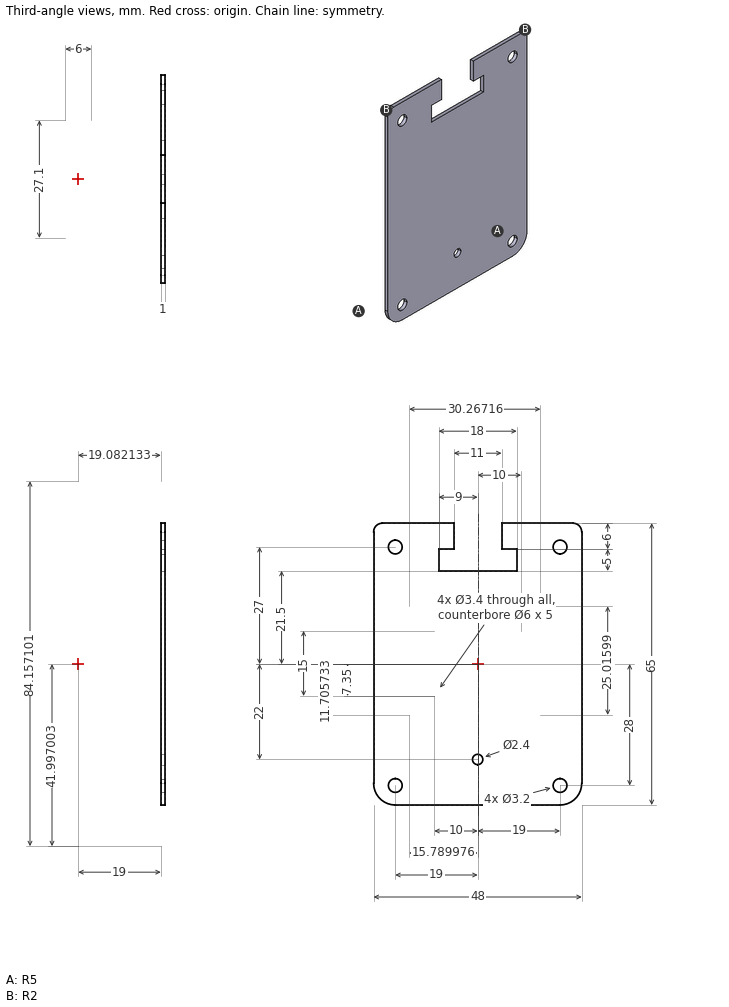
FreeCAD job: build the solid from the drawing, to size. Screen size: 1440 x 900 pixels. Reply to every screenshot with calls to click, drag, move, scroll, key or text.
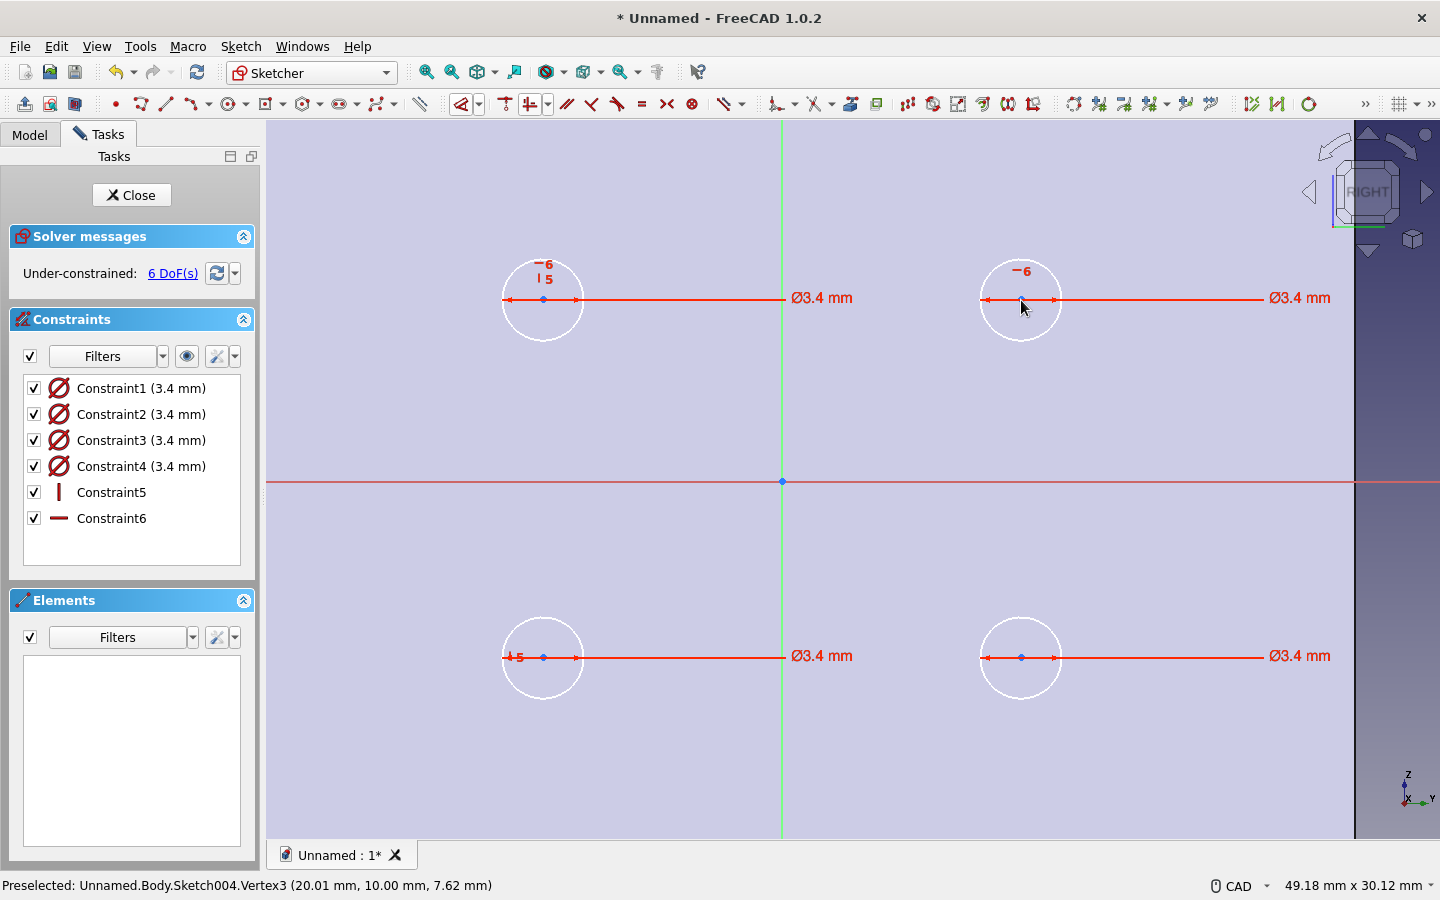
click(1021, 300)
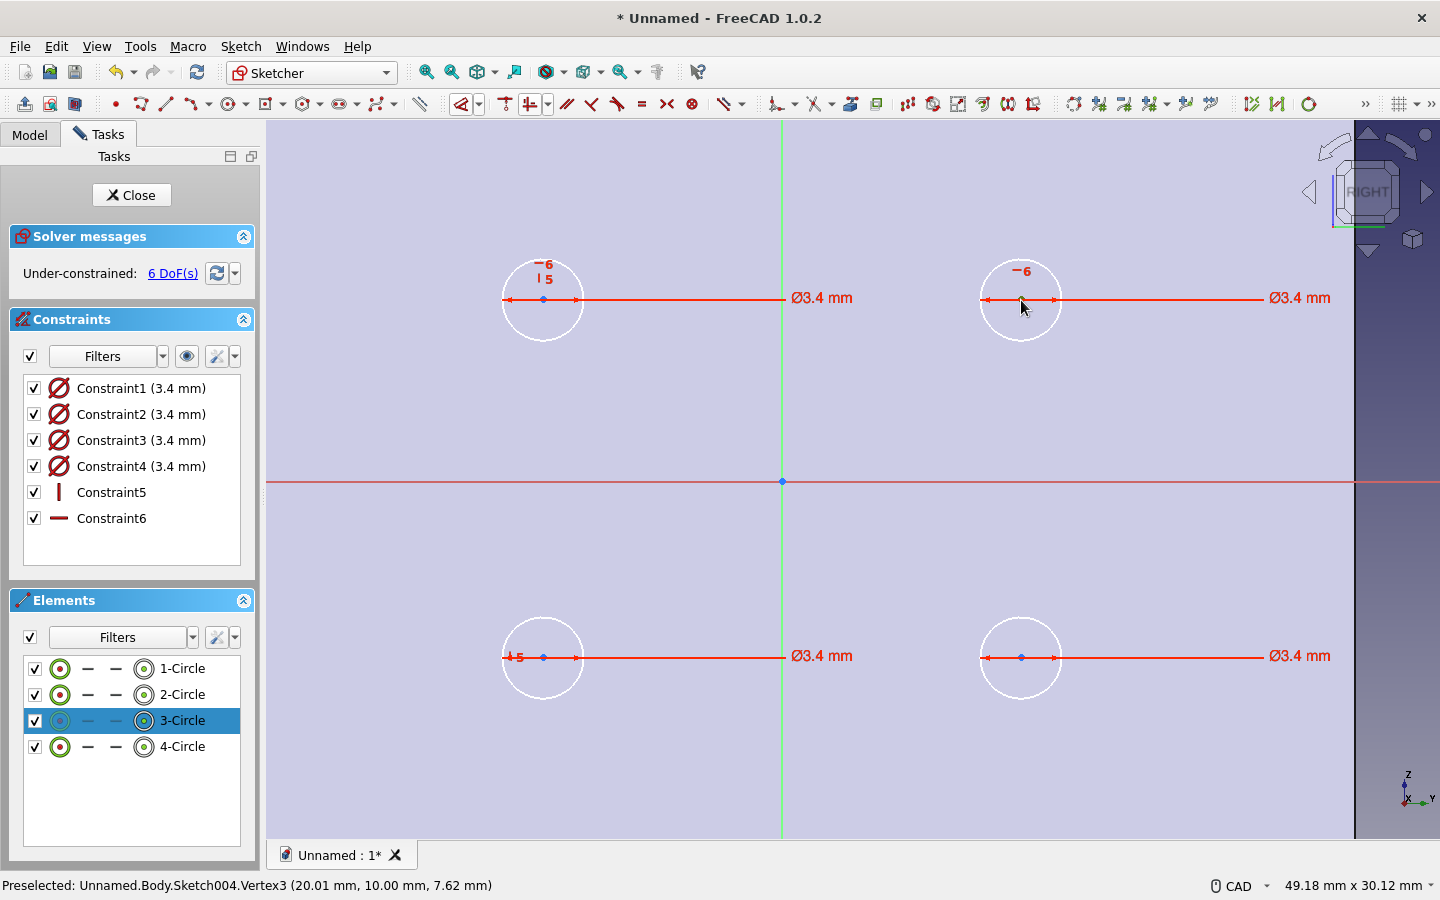
click(1021, 658)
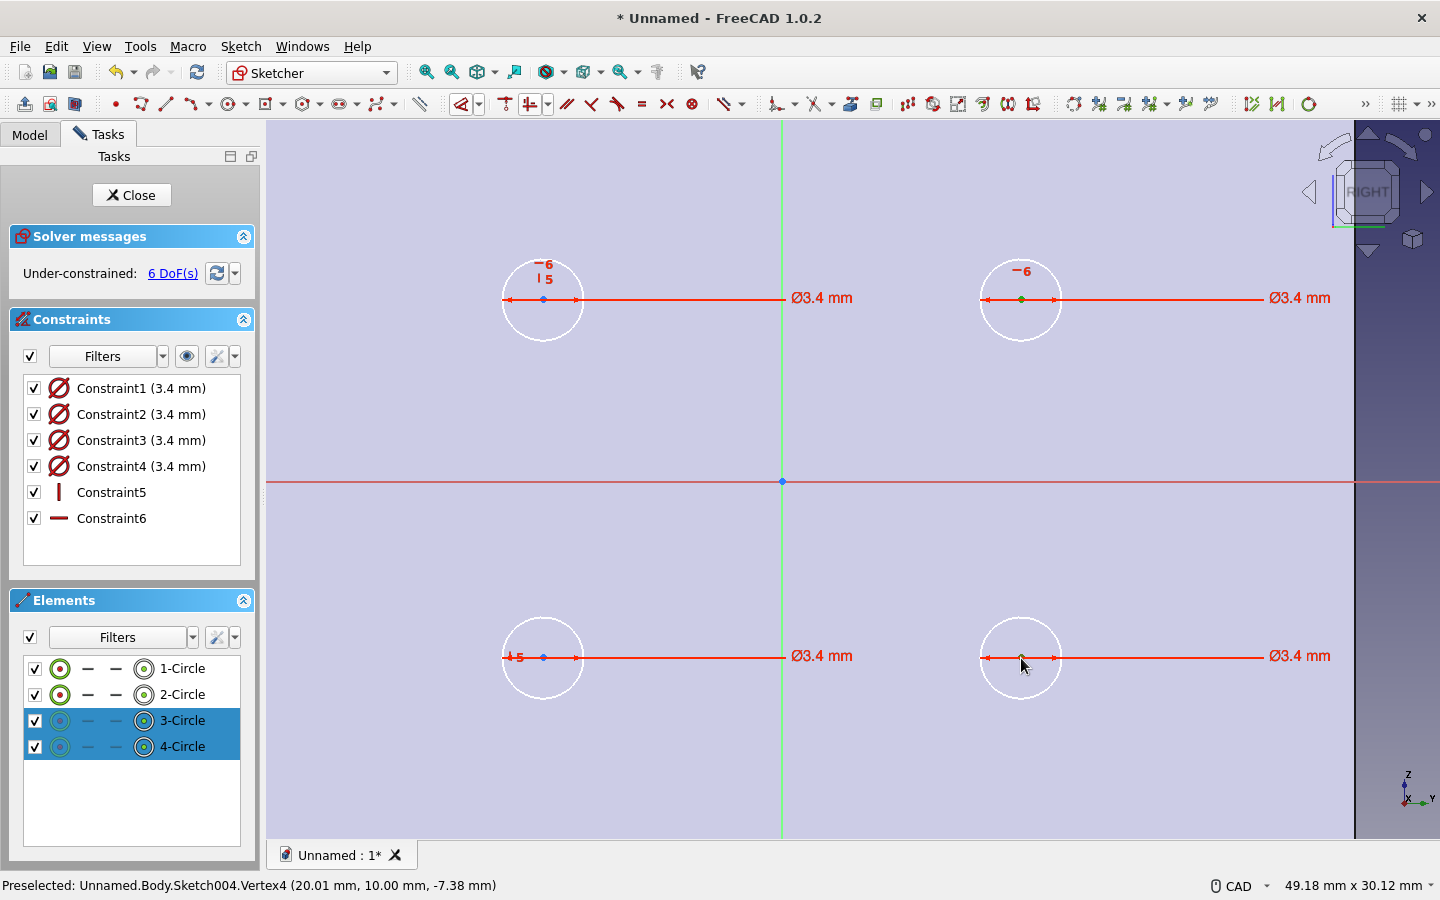
key(v)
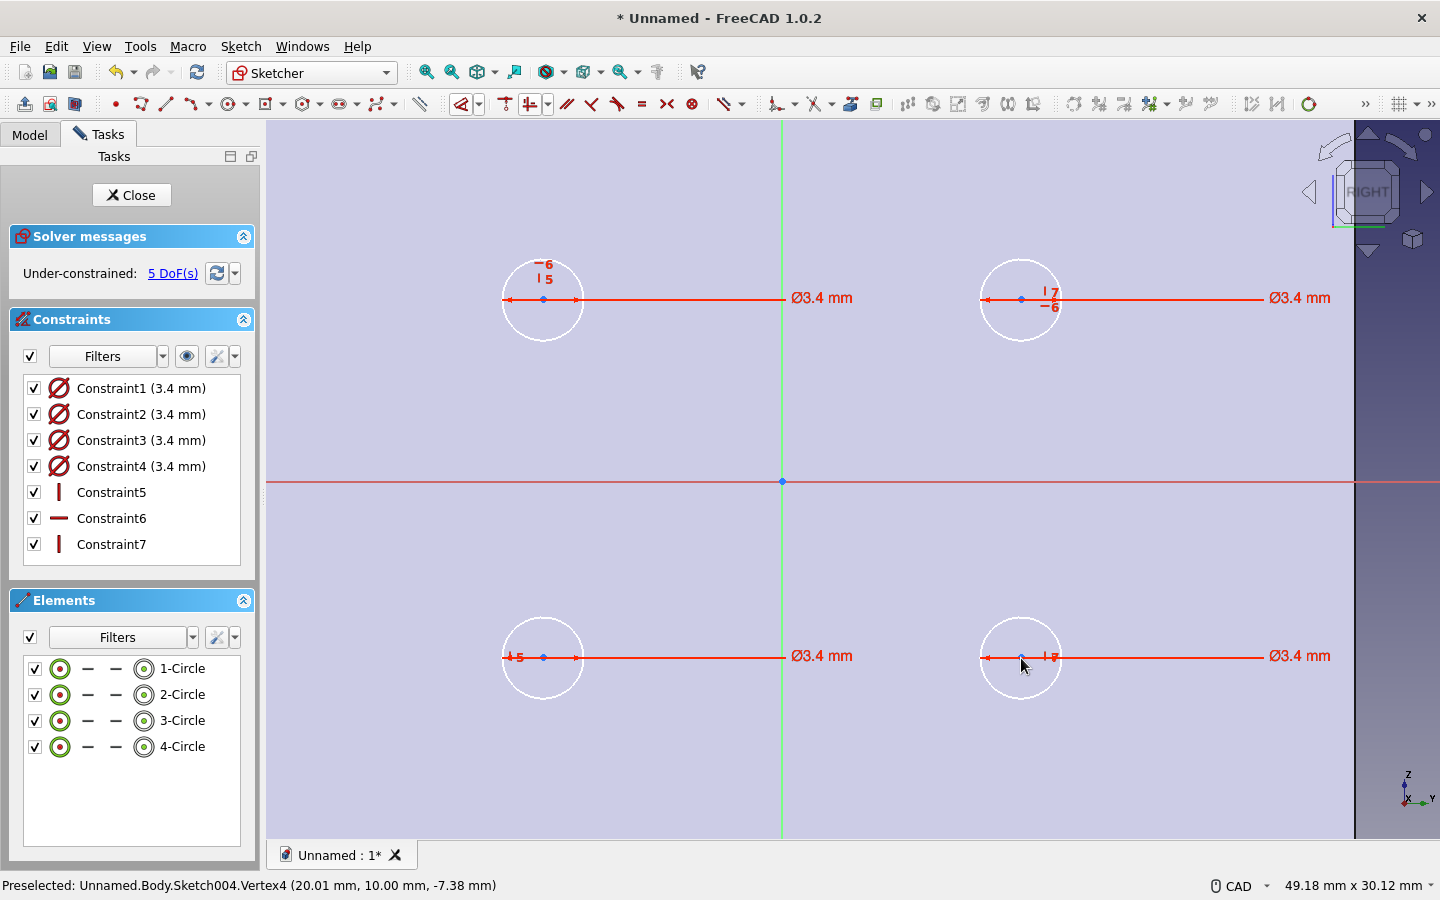
click(543, 658)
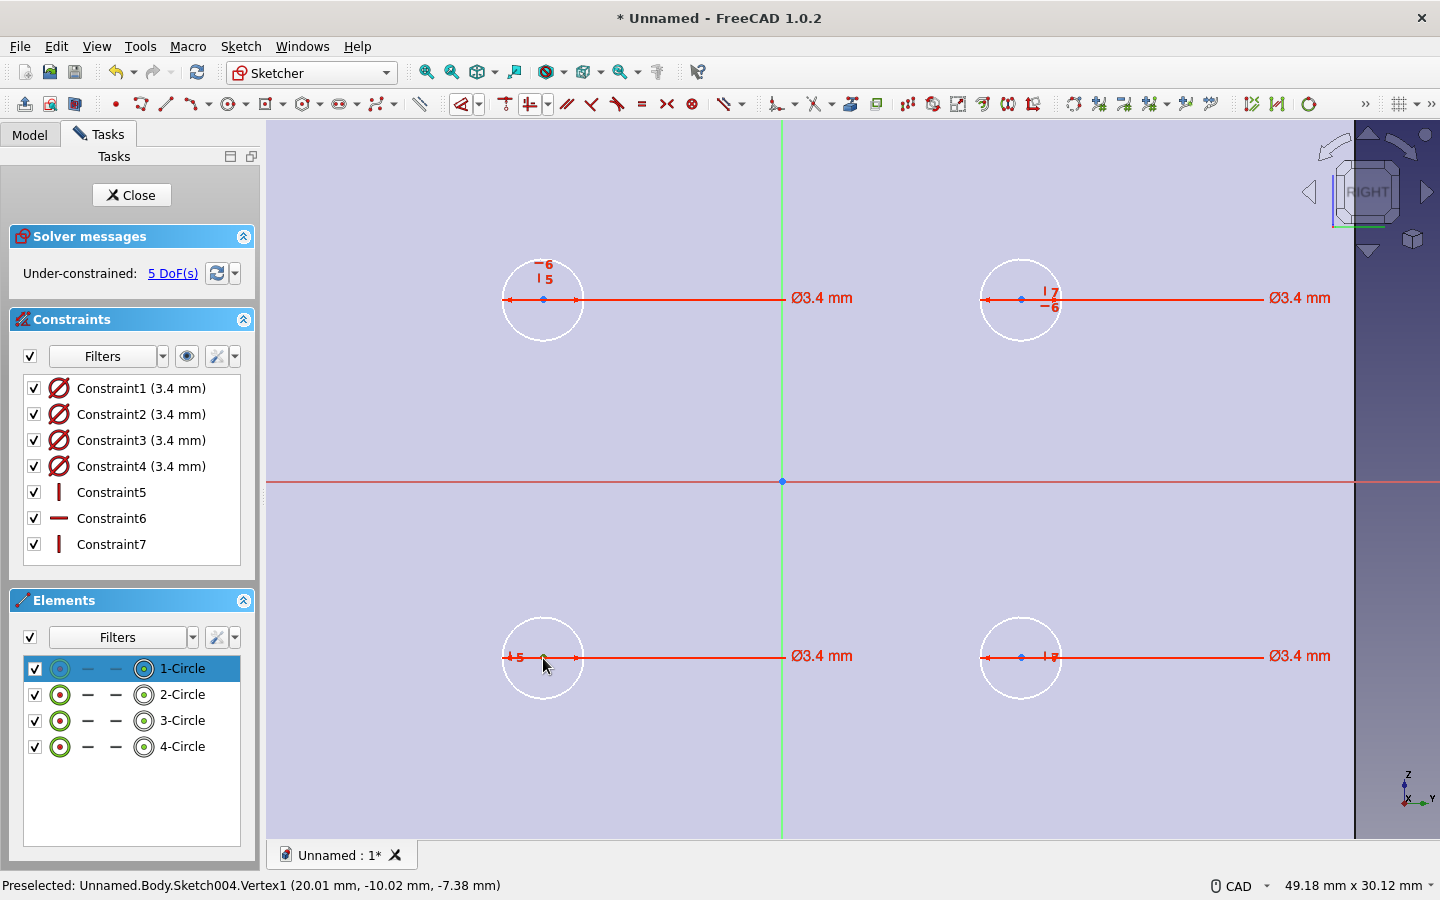
click(1021, 658)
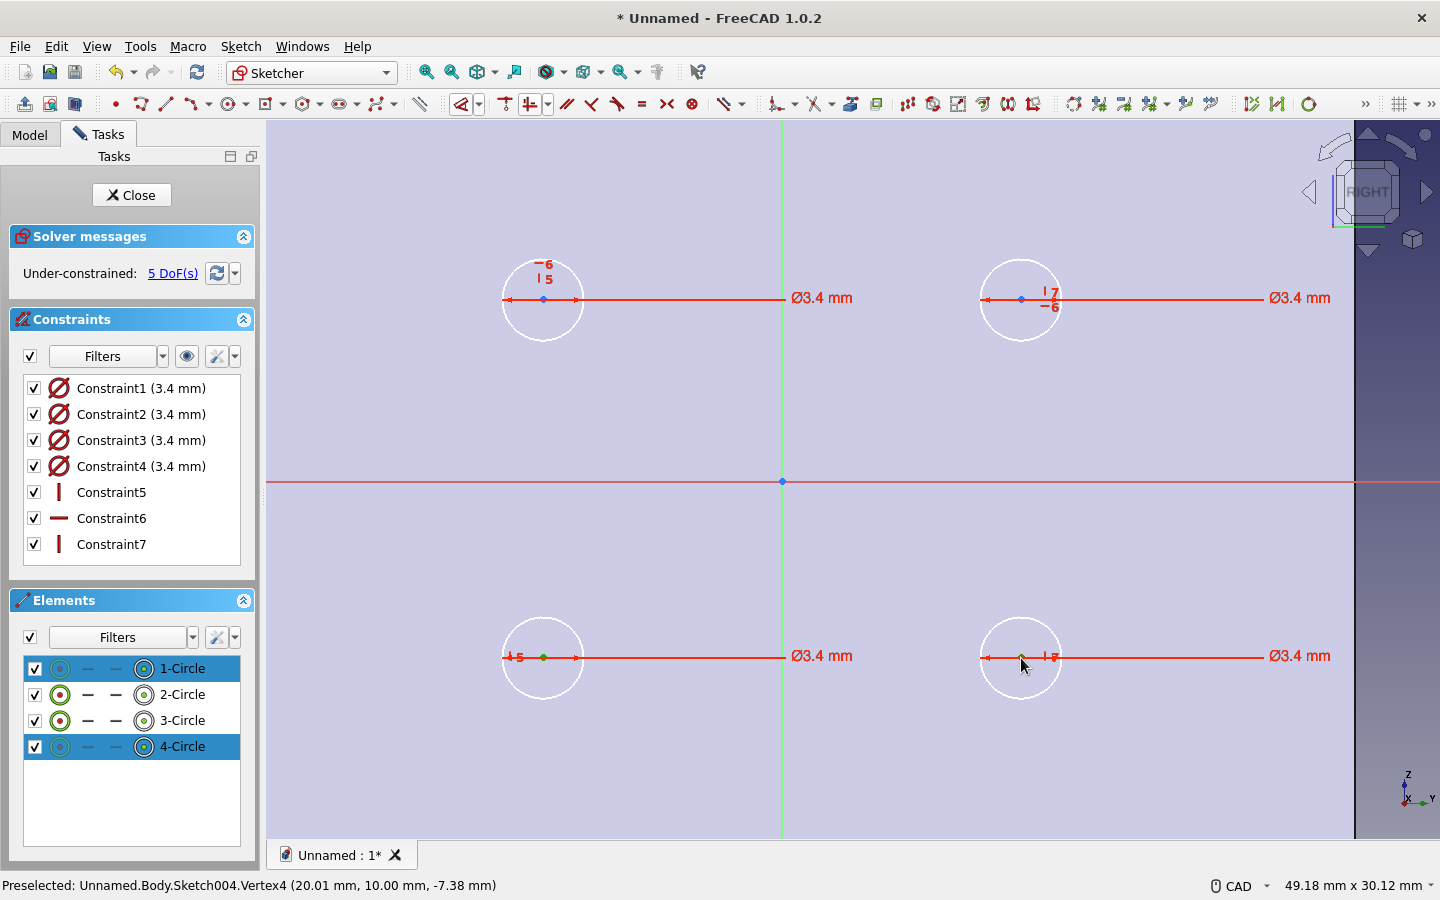
key(h)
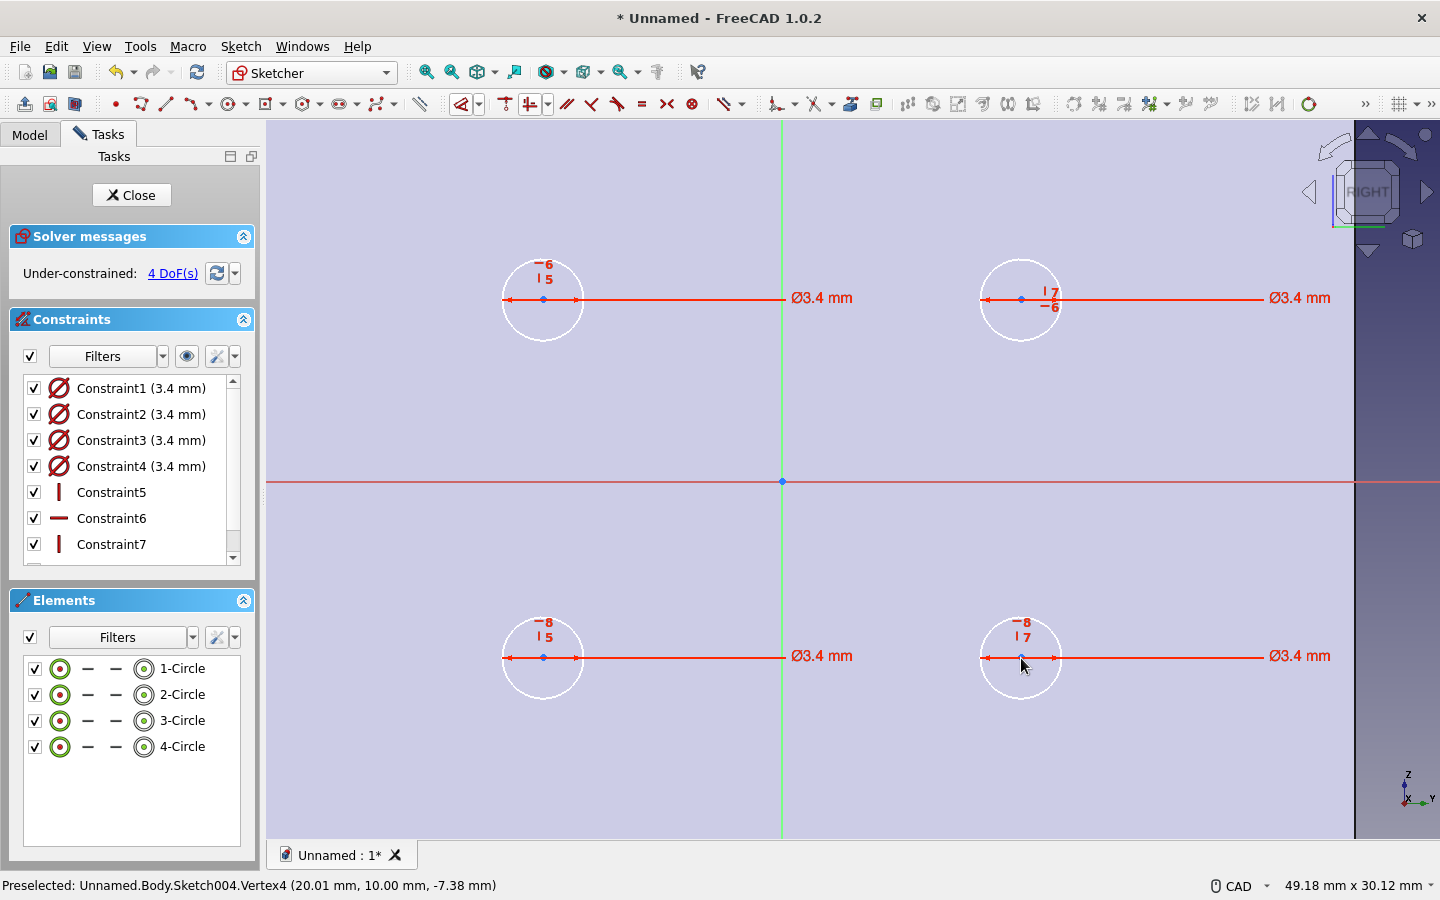
click(543, 658)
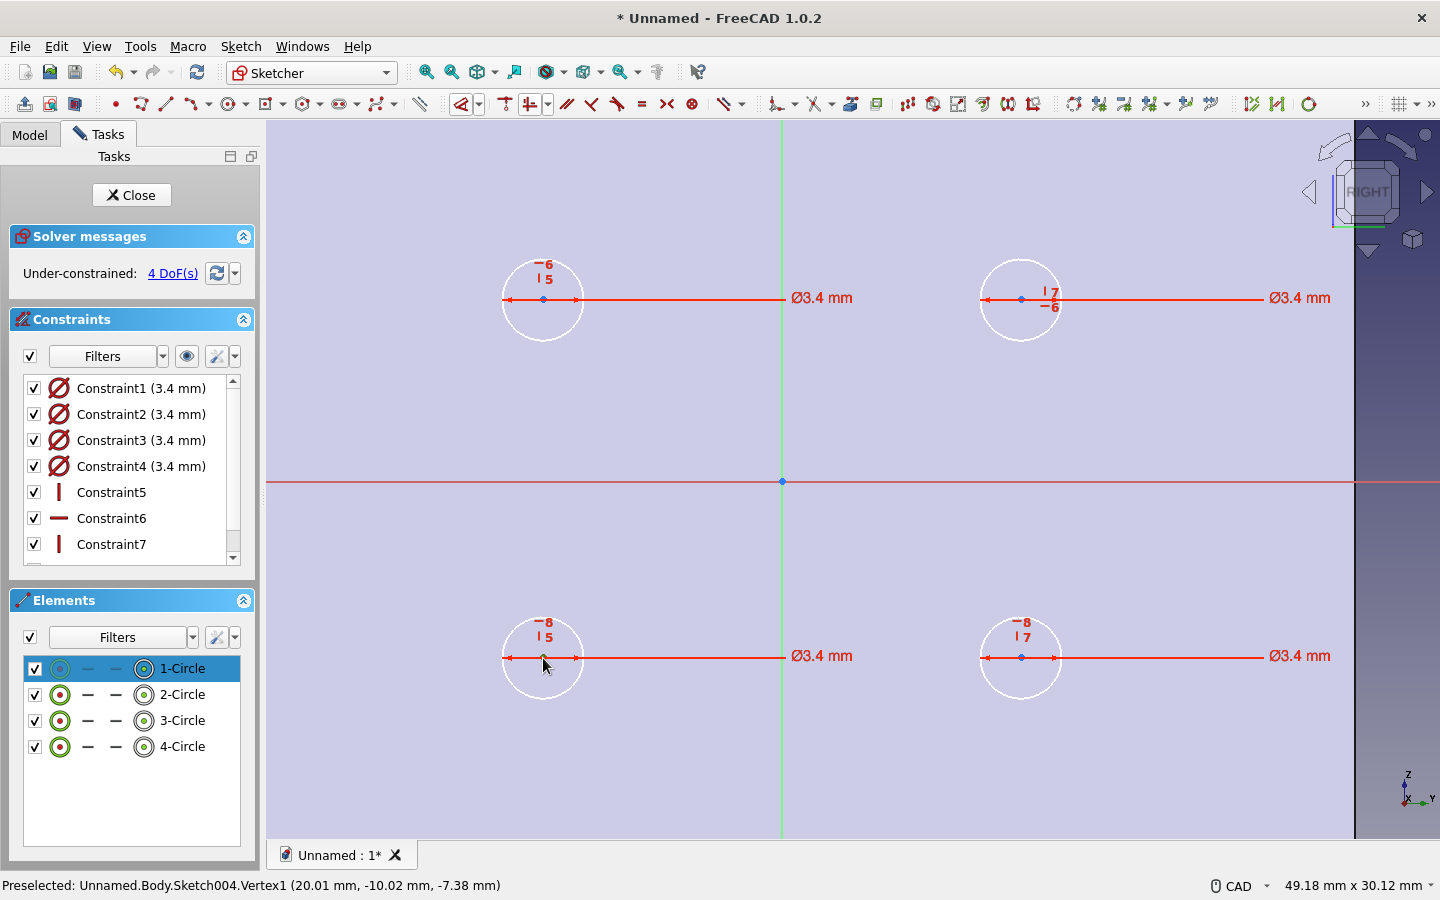
click(478, 104)